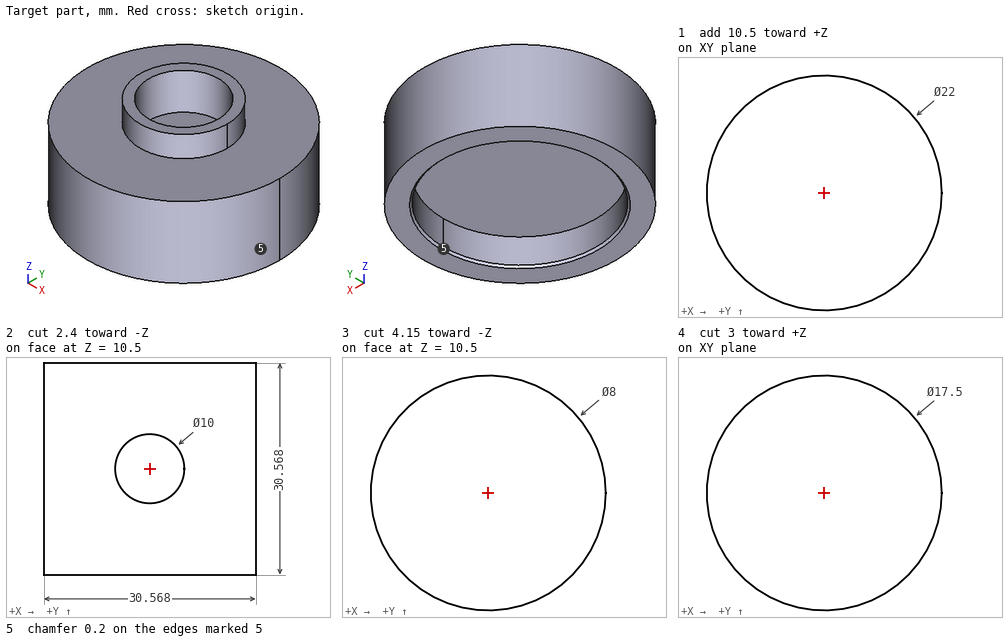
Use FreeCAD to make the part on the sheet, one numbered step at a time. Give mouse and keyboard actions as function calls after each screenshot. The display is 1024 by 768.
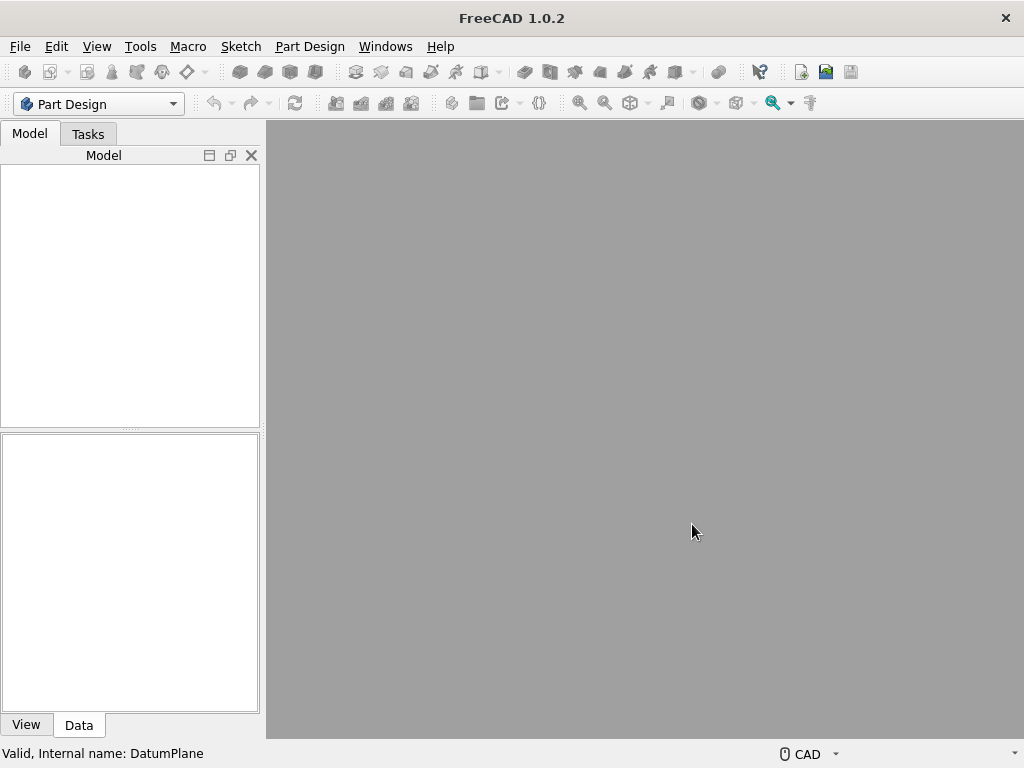
click(801, 72)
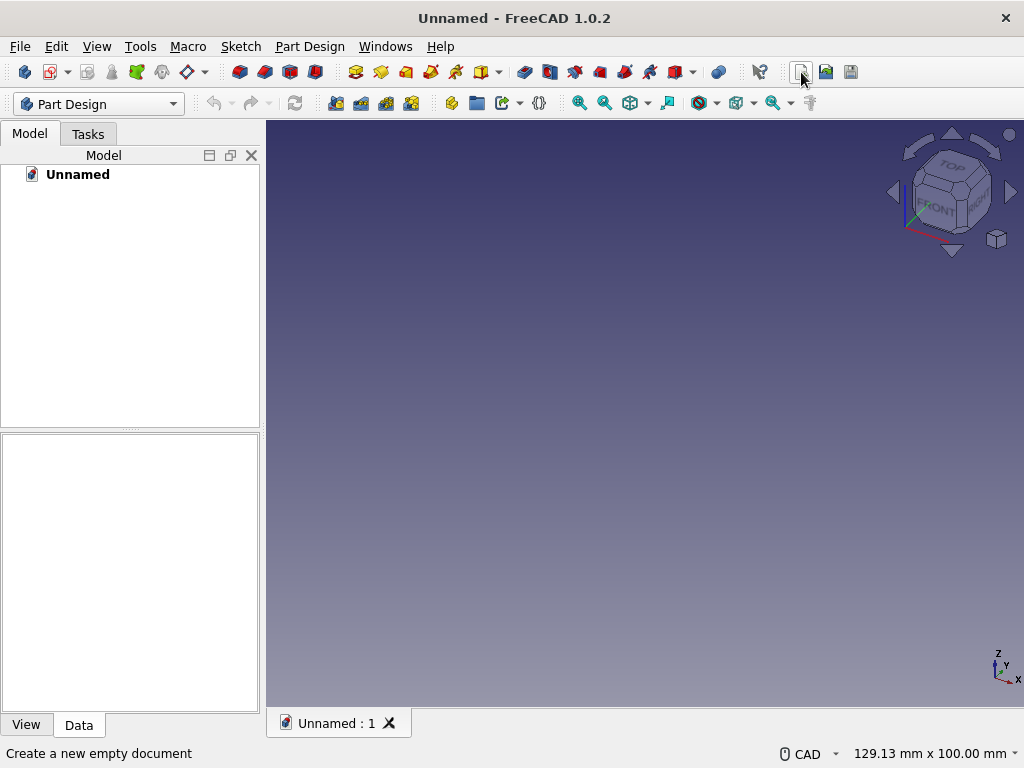
click(50, 72)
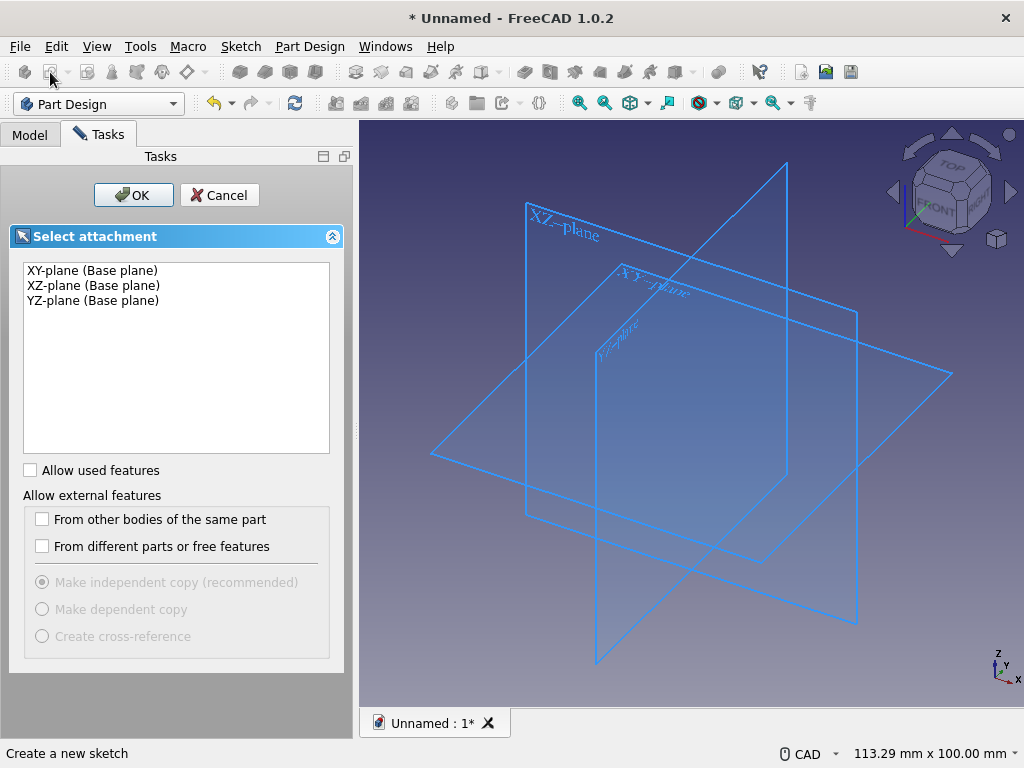
click(84, 270)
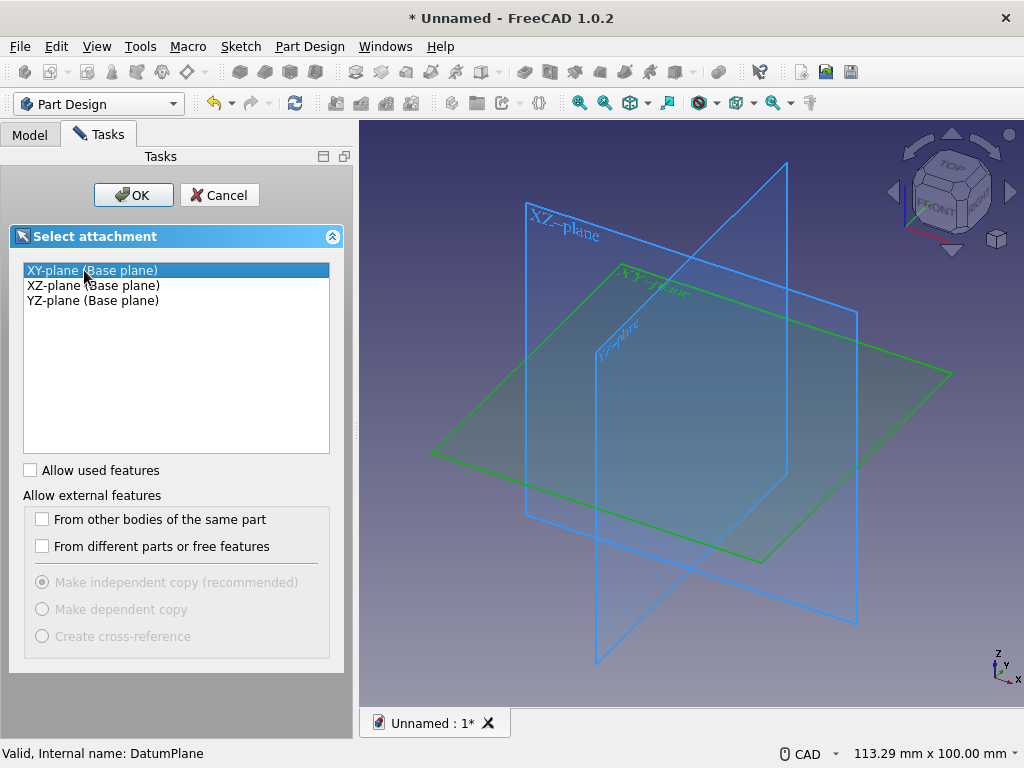
click(134, 195)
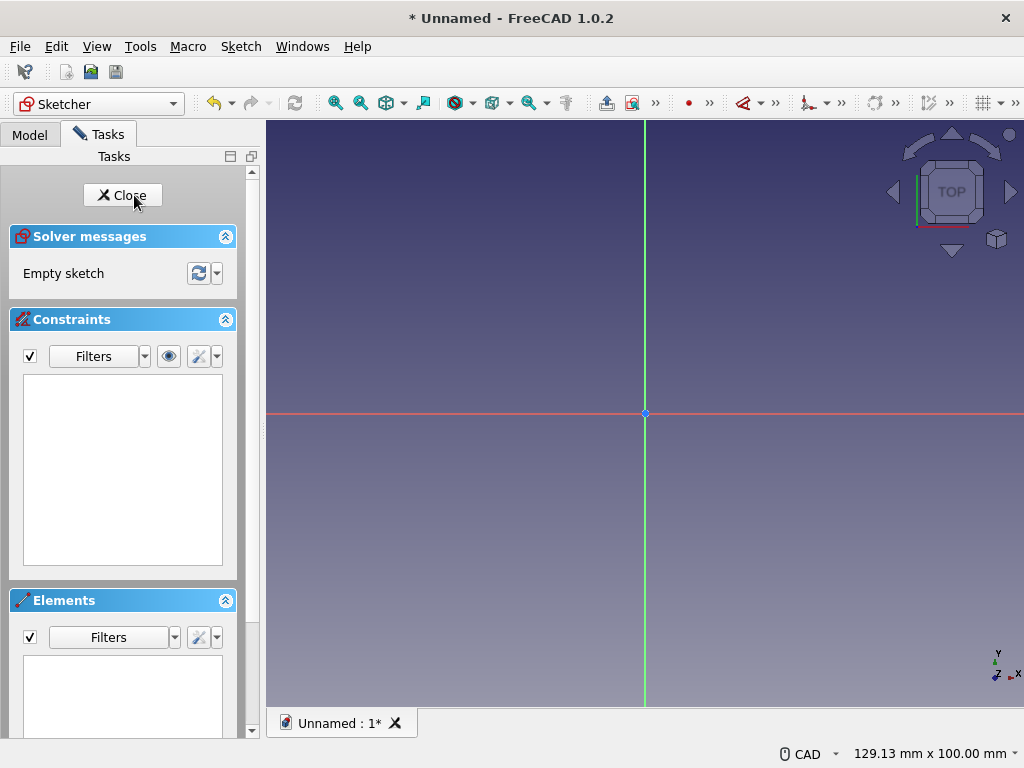
scroll(685, 414, up, 5)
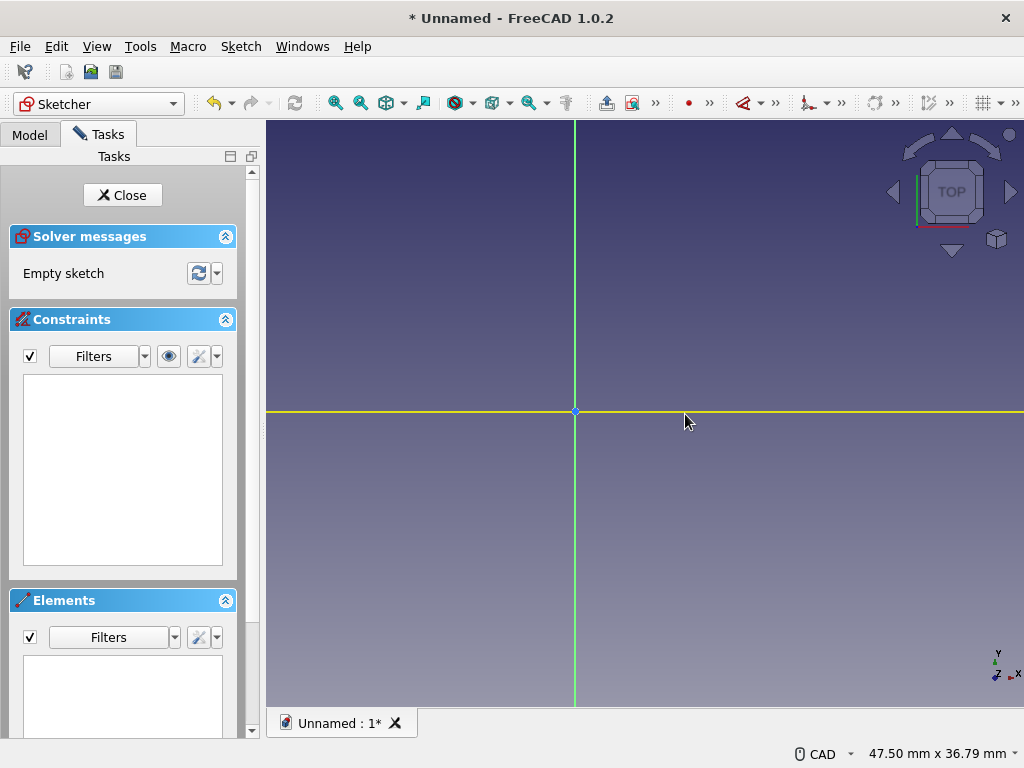
key(g)
key(c)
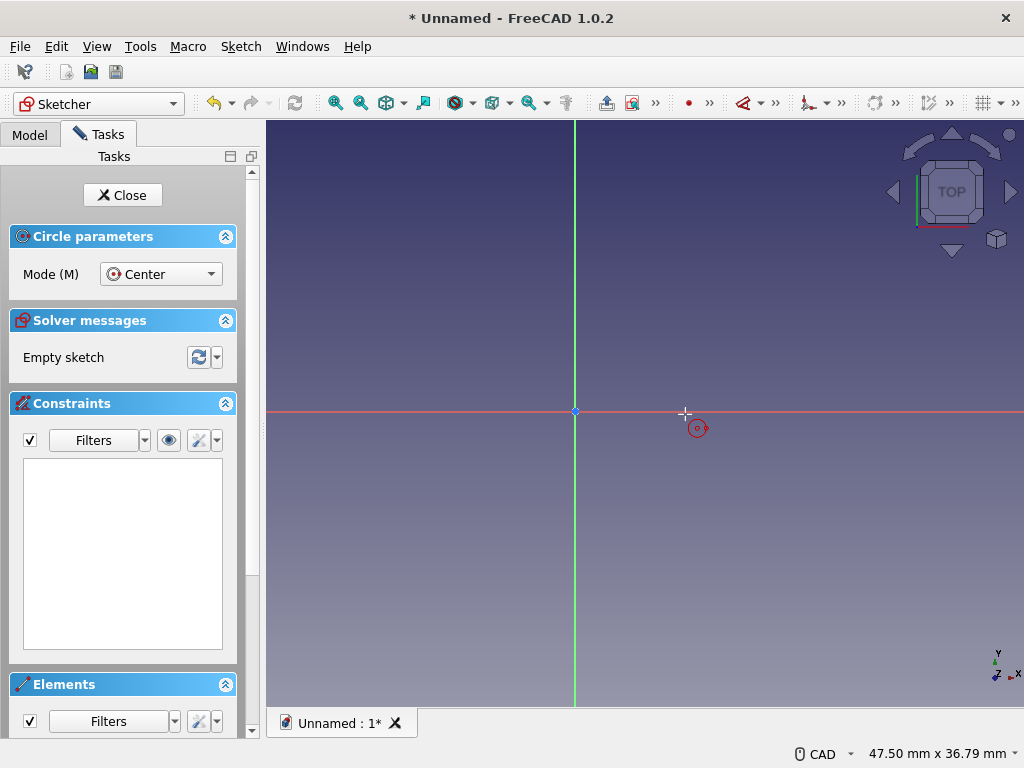
click(575, 412)
move(699, 288)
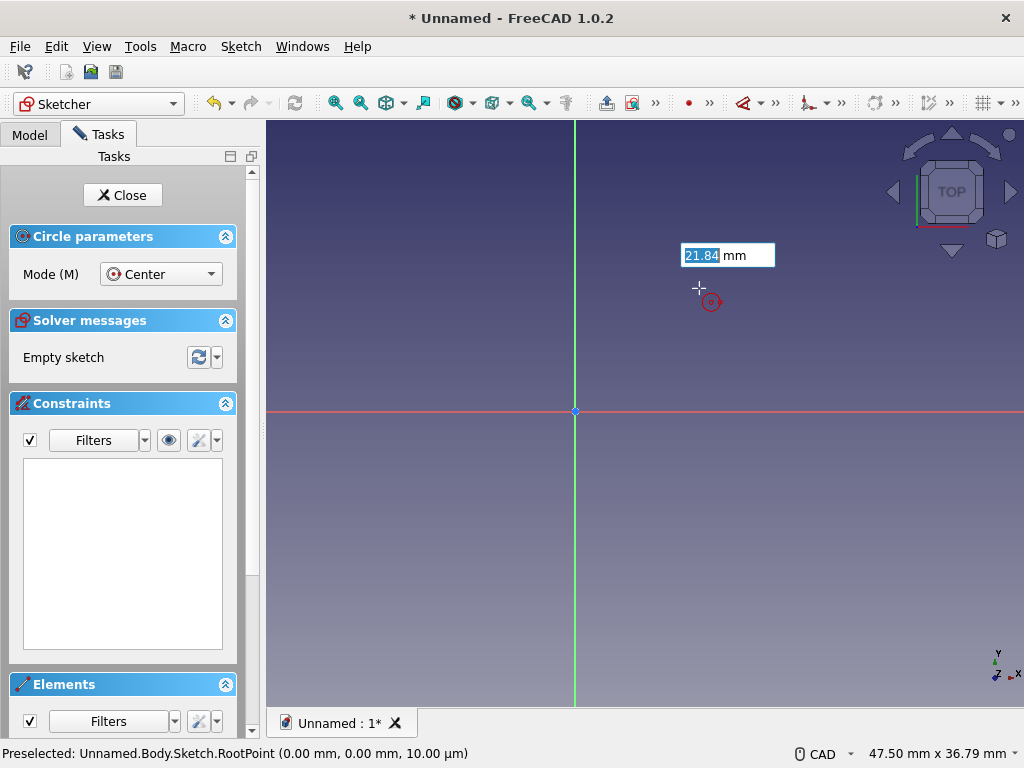
text(22)
key(Return)
key(Escape)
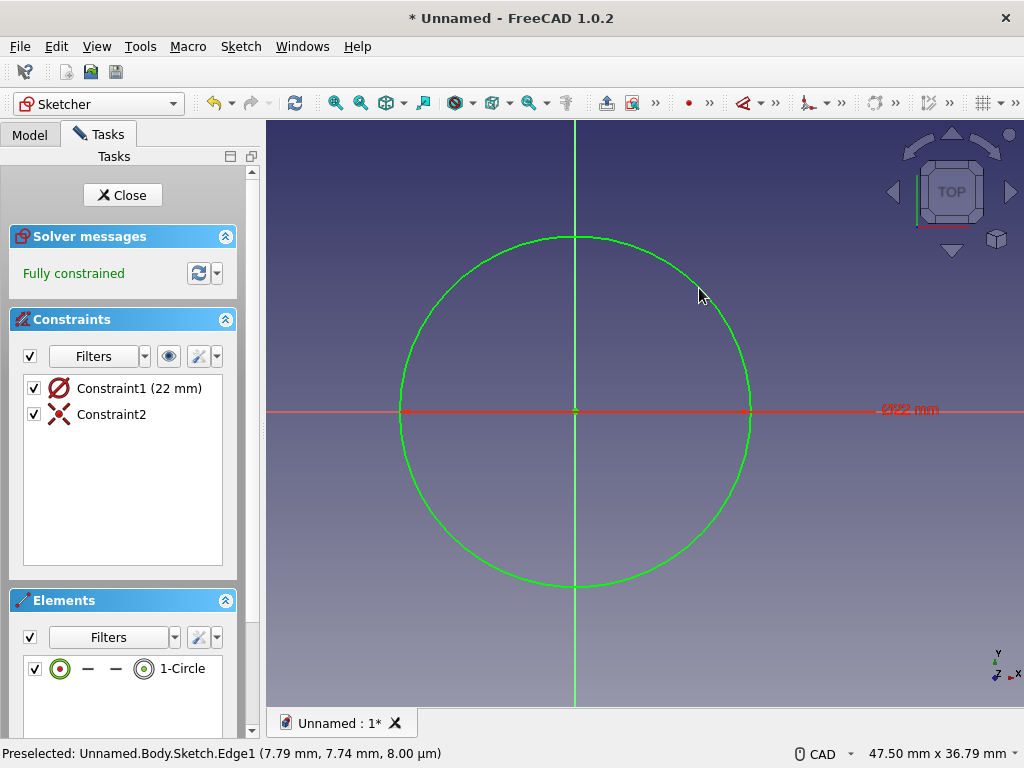
click(123, 195)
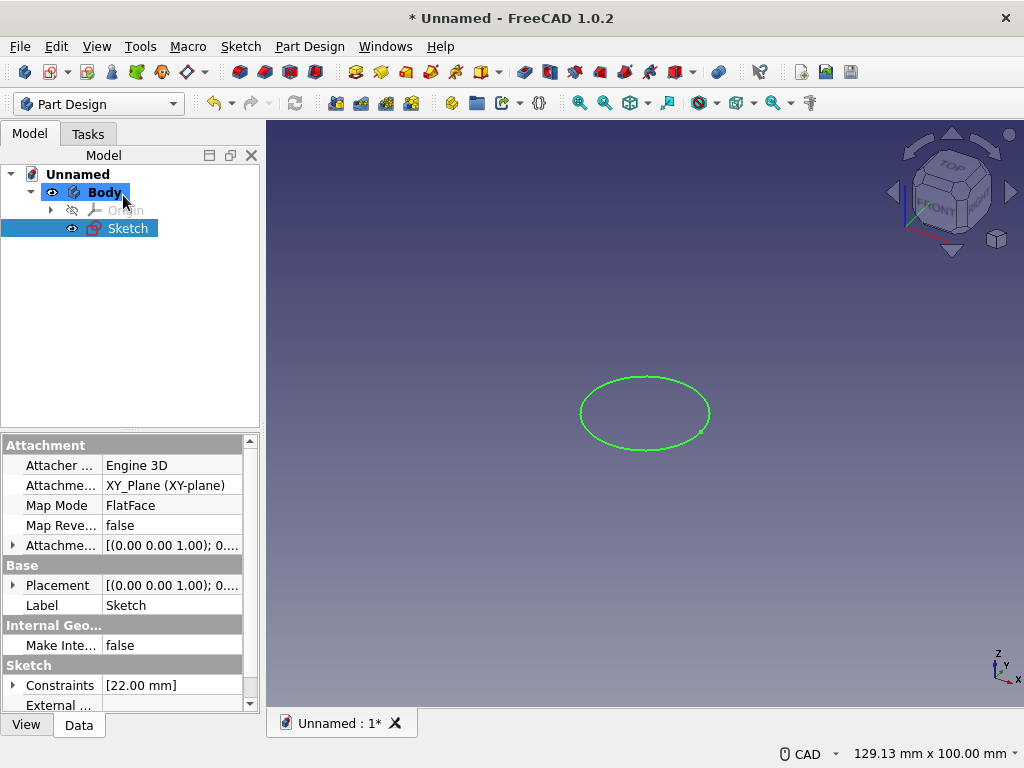
click(356, 72)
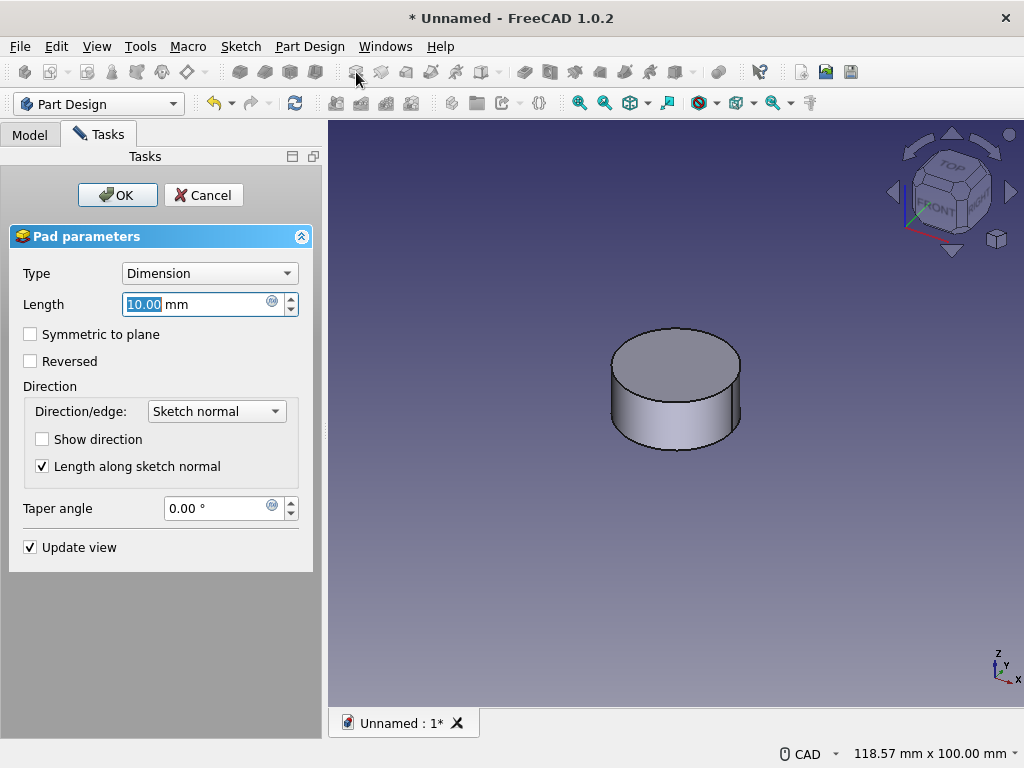
text(10.5)
key(Tab)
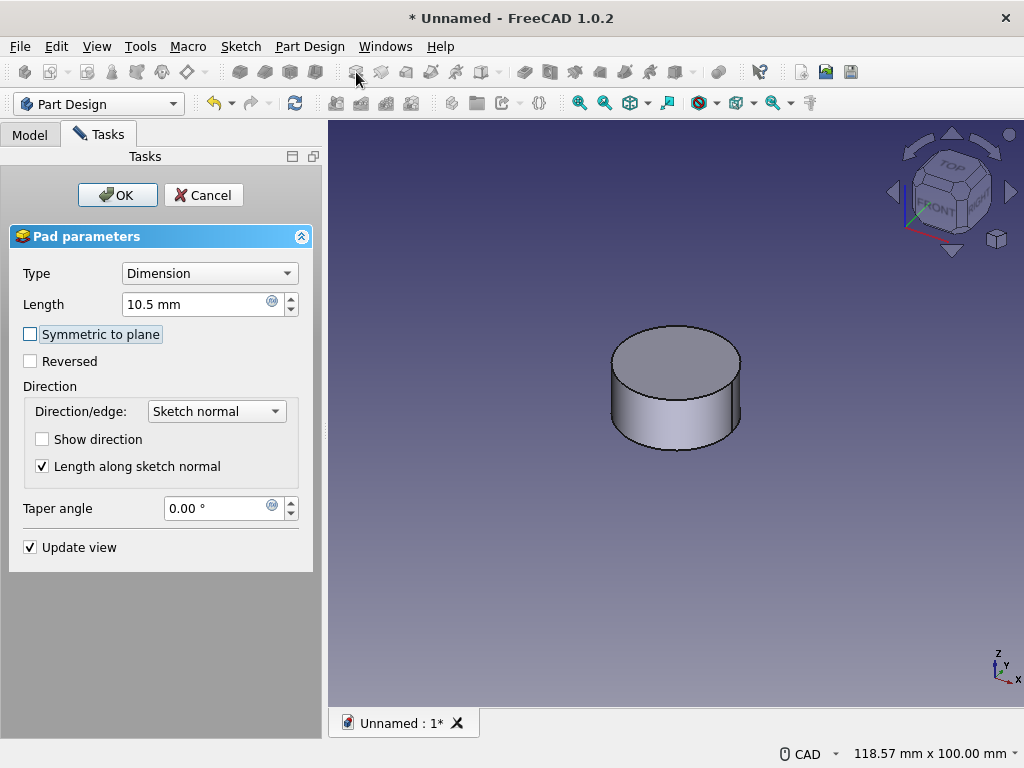
click(118, 195)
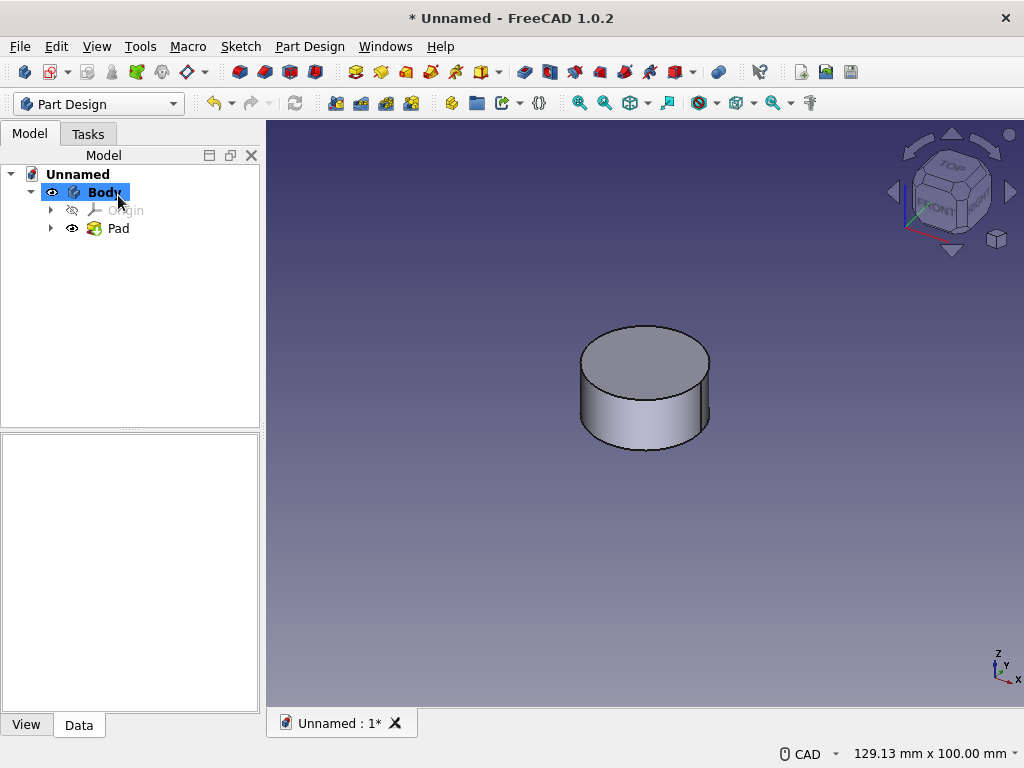
click(580, 104)